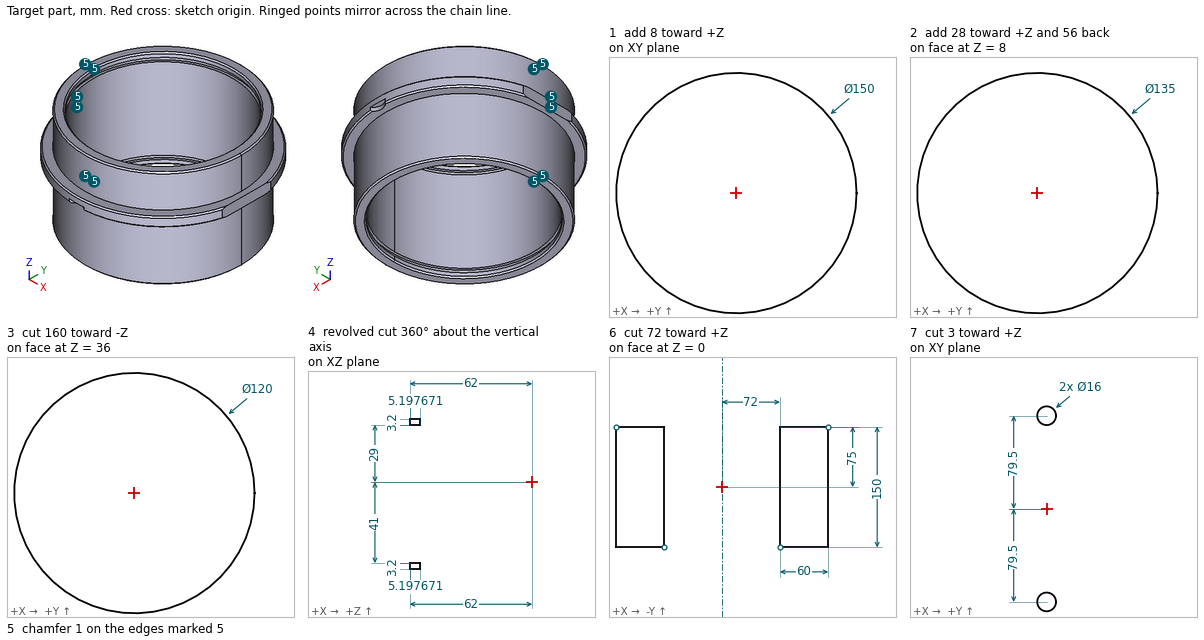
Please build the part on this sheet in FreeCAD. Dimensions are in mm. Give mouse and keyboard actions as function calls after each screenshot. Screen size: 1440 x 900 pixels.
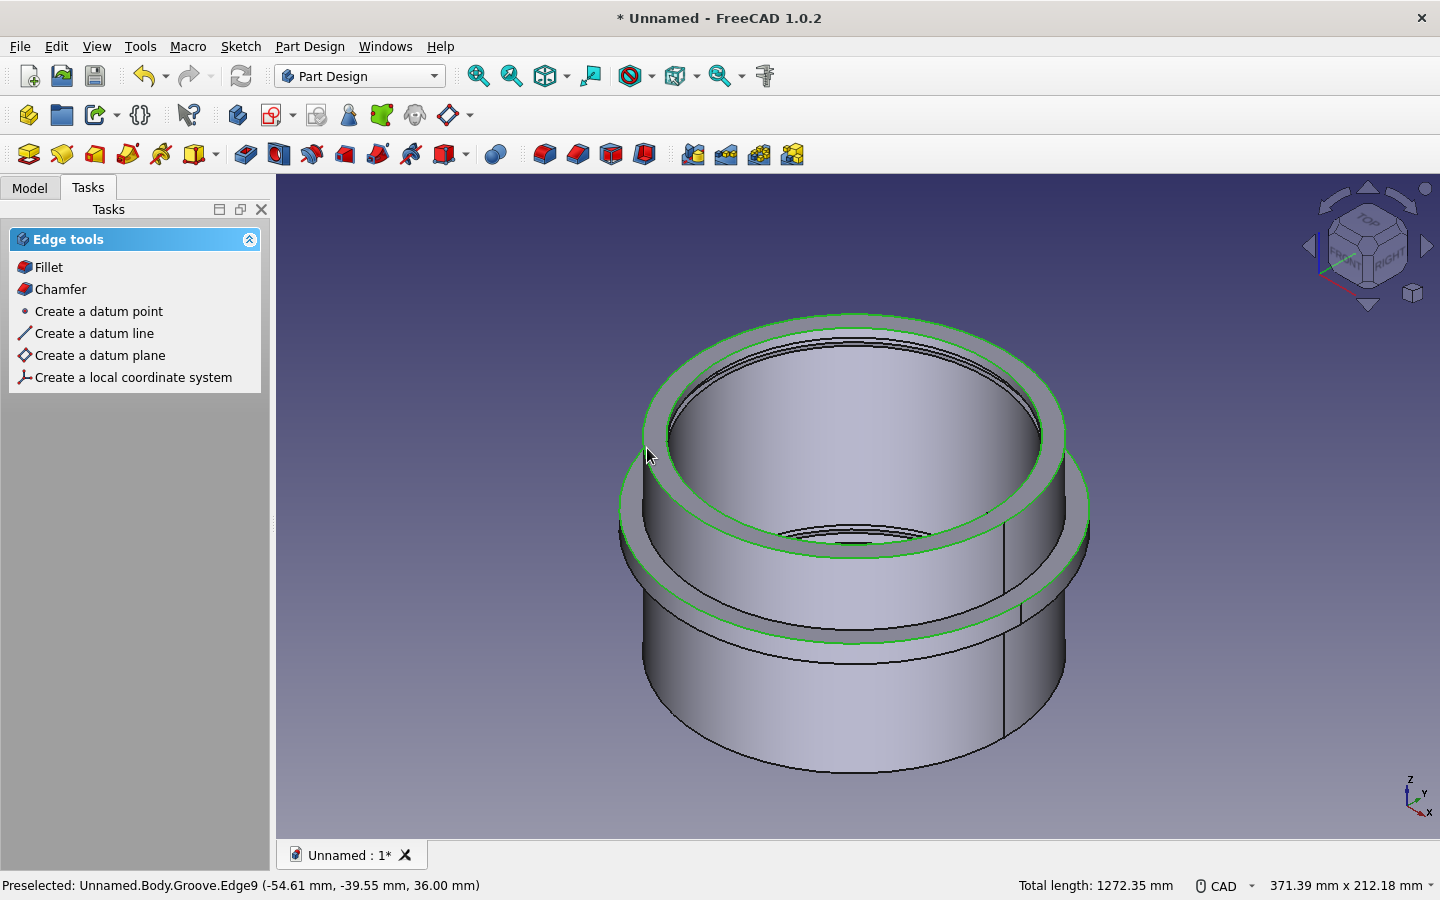
key(v)
key(f)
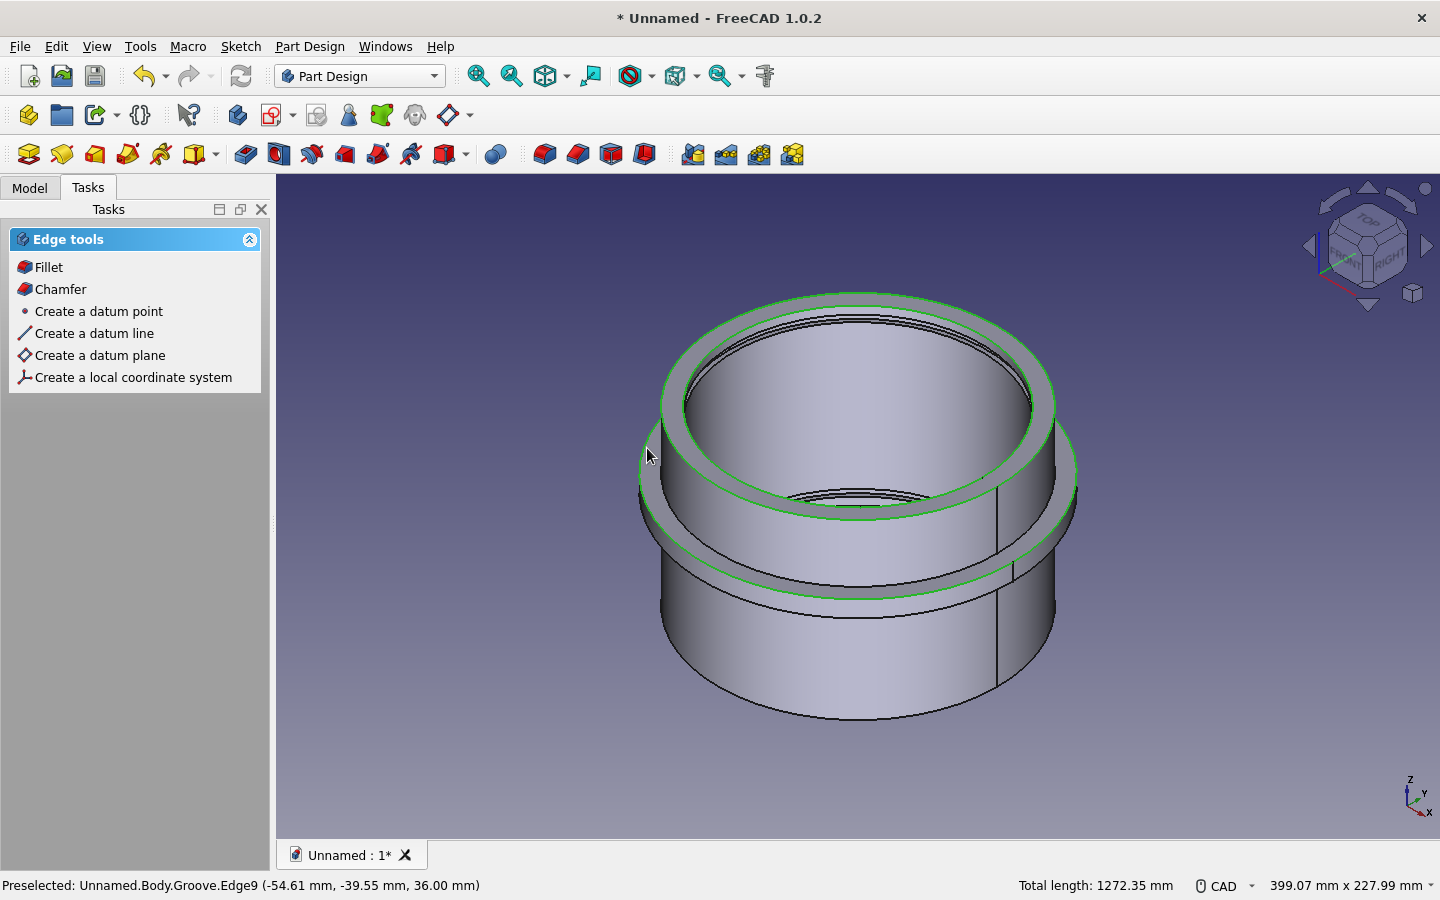
click(663, 549, ctrl)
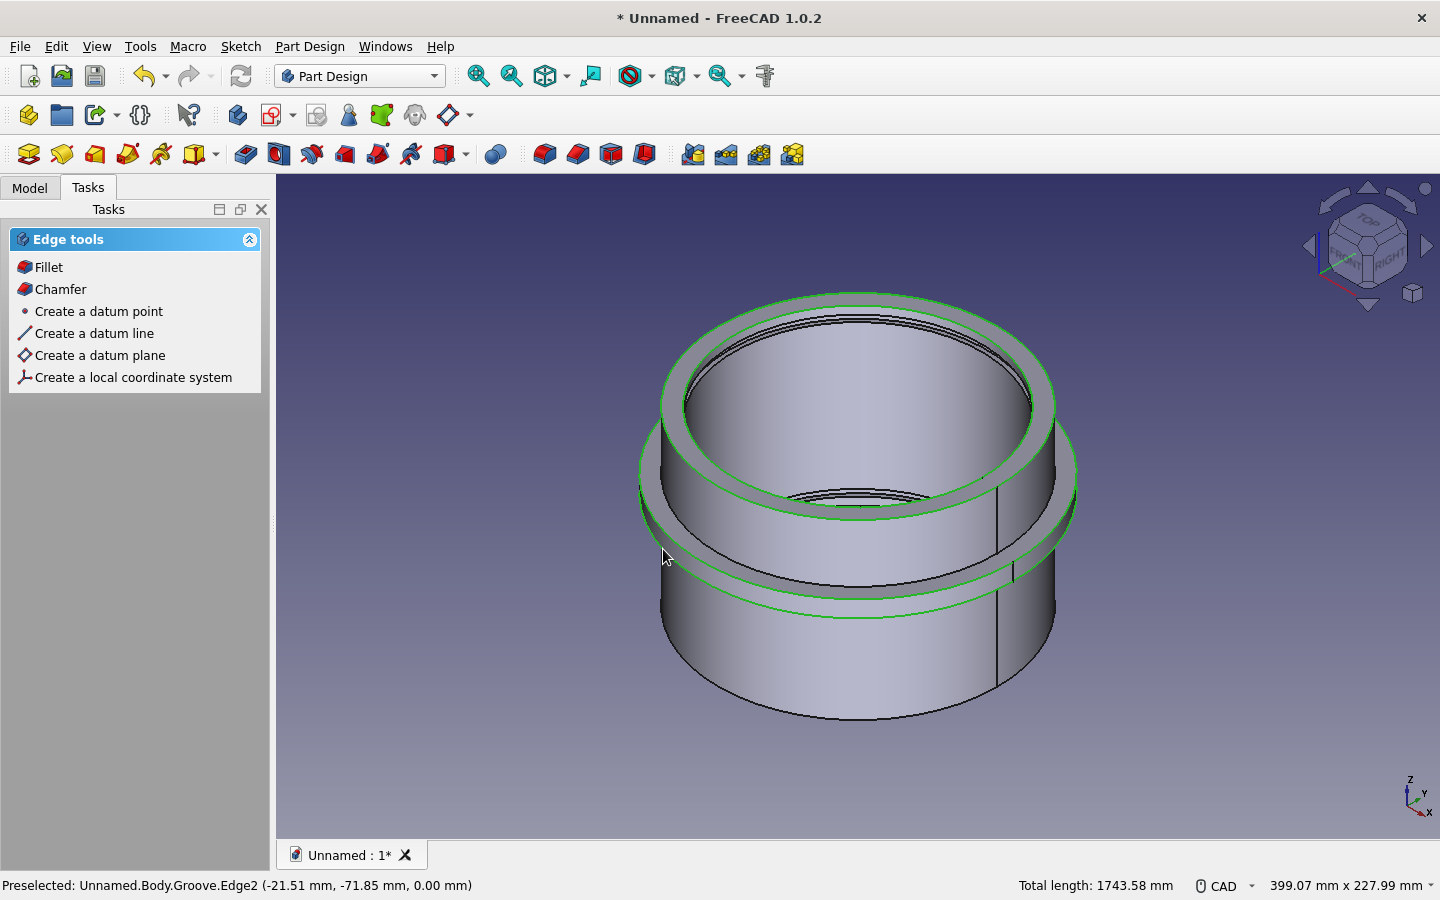
key(2)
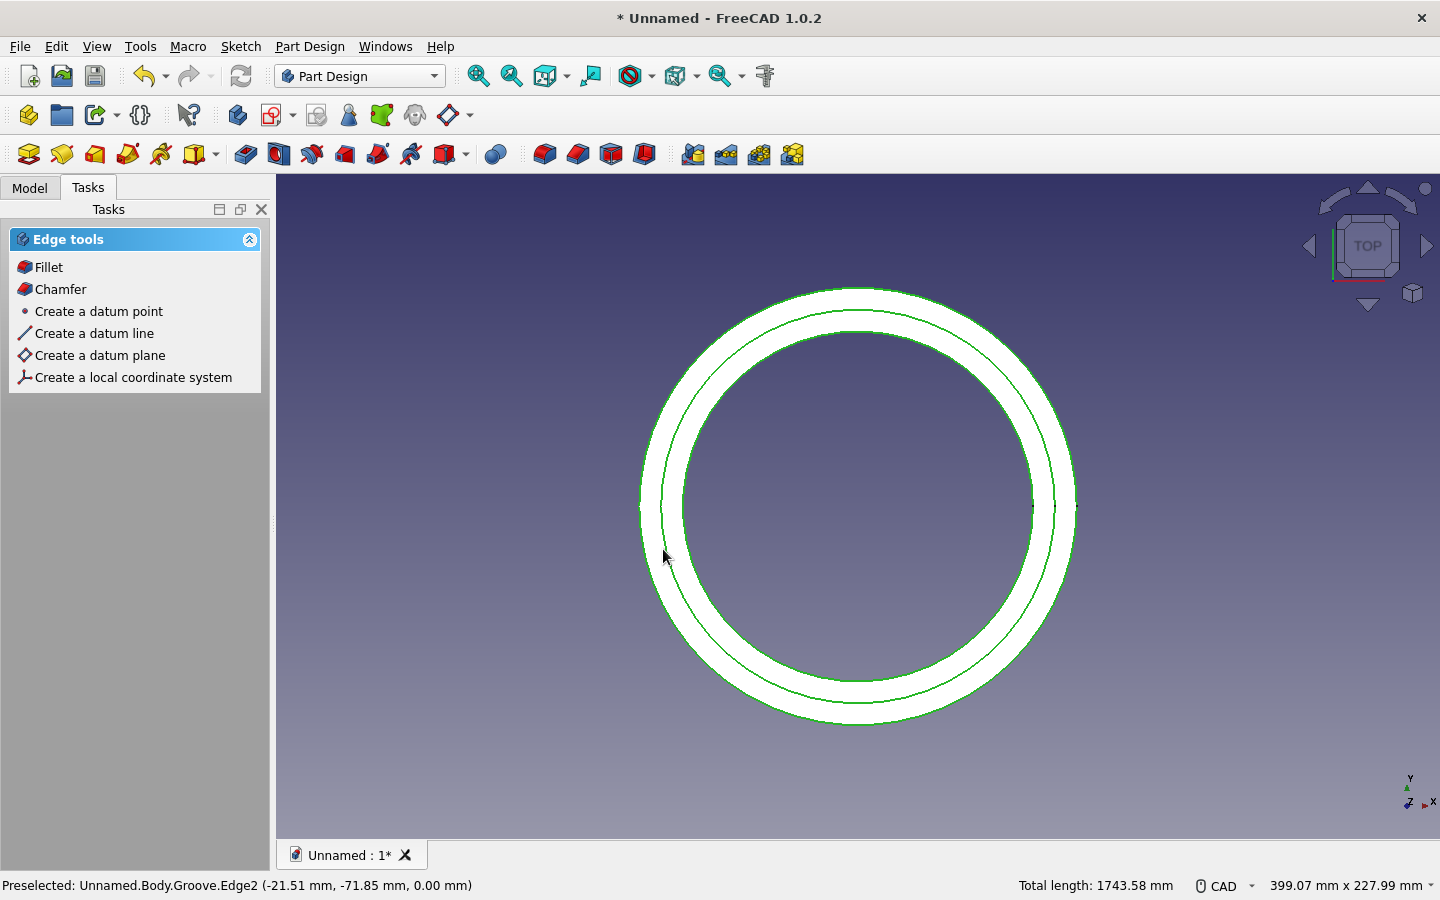
key(1)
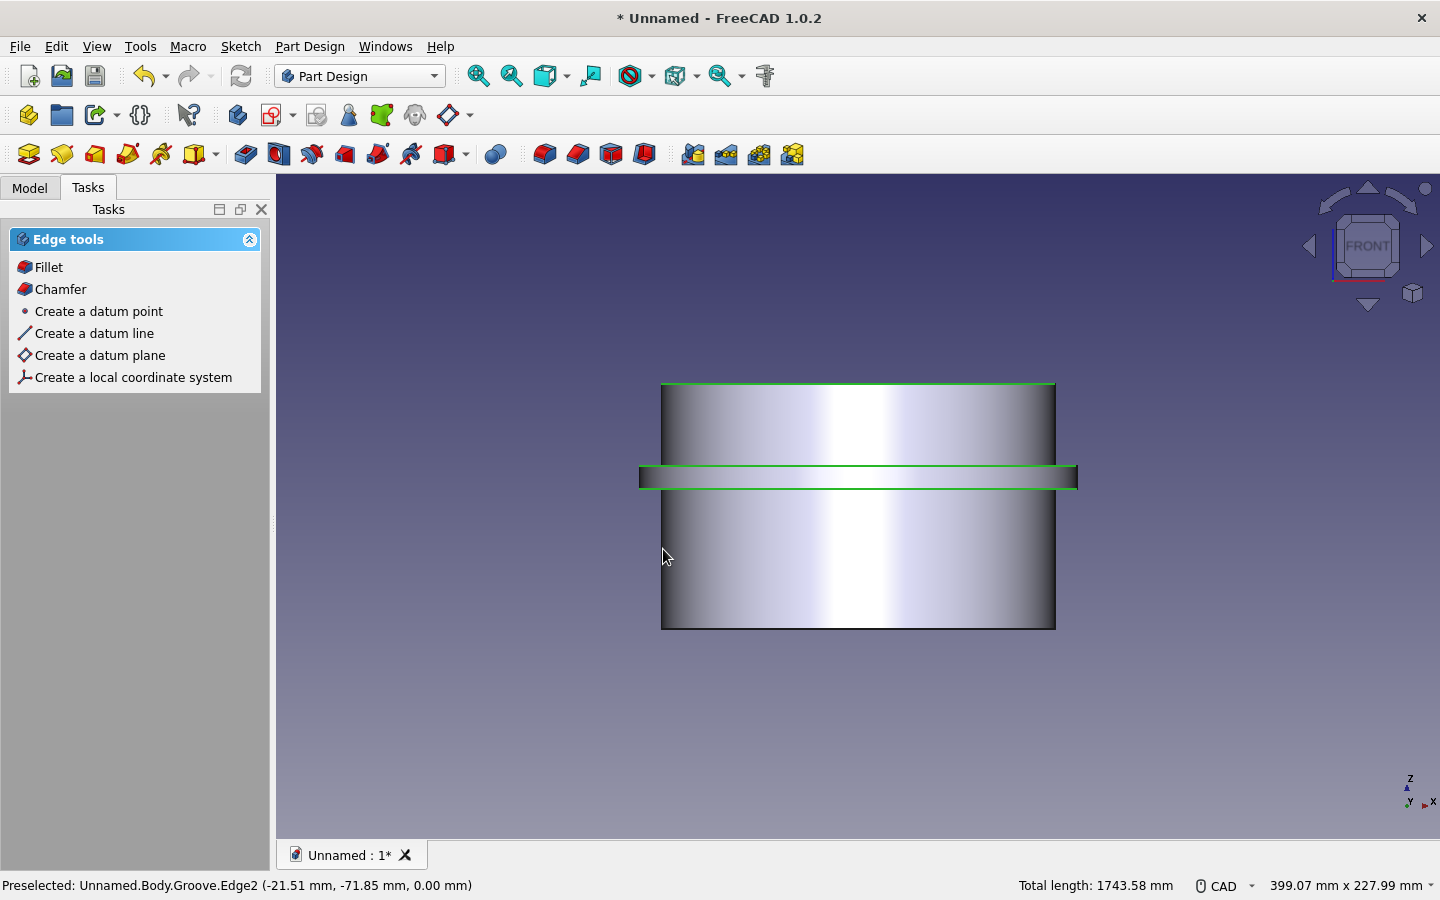
click(479, 76)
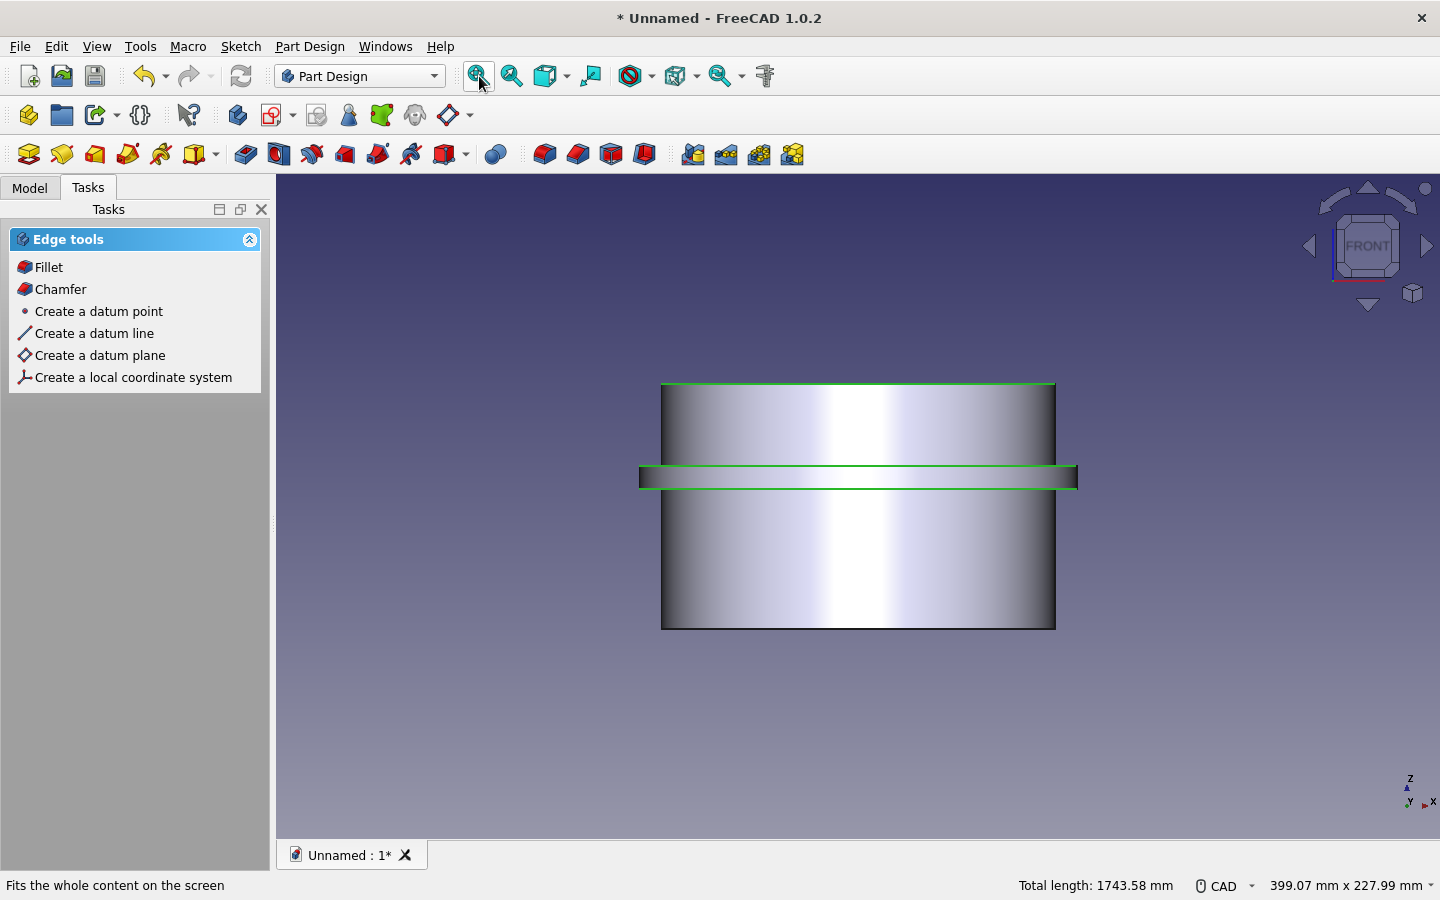
click(699, 628, ctrl)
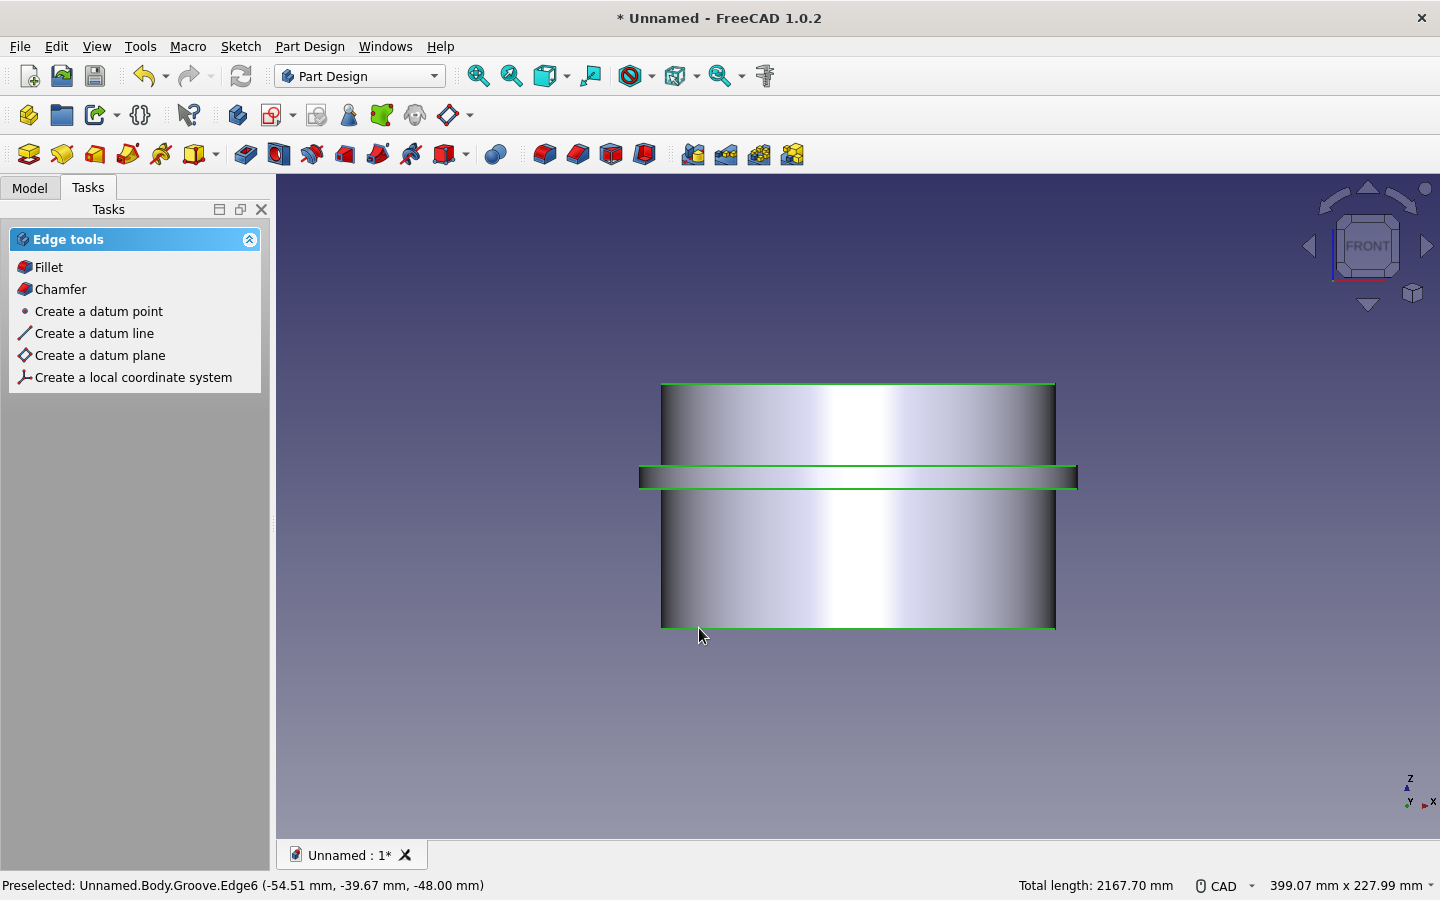
key(3)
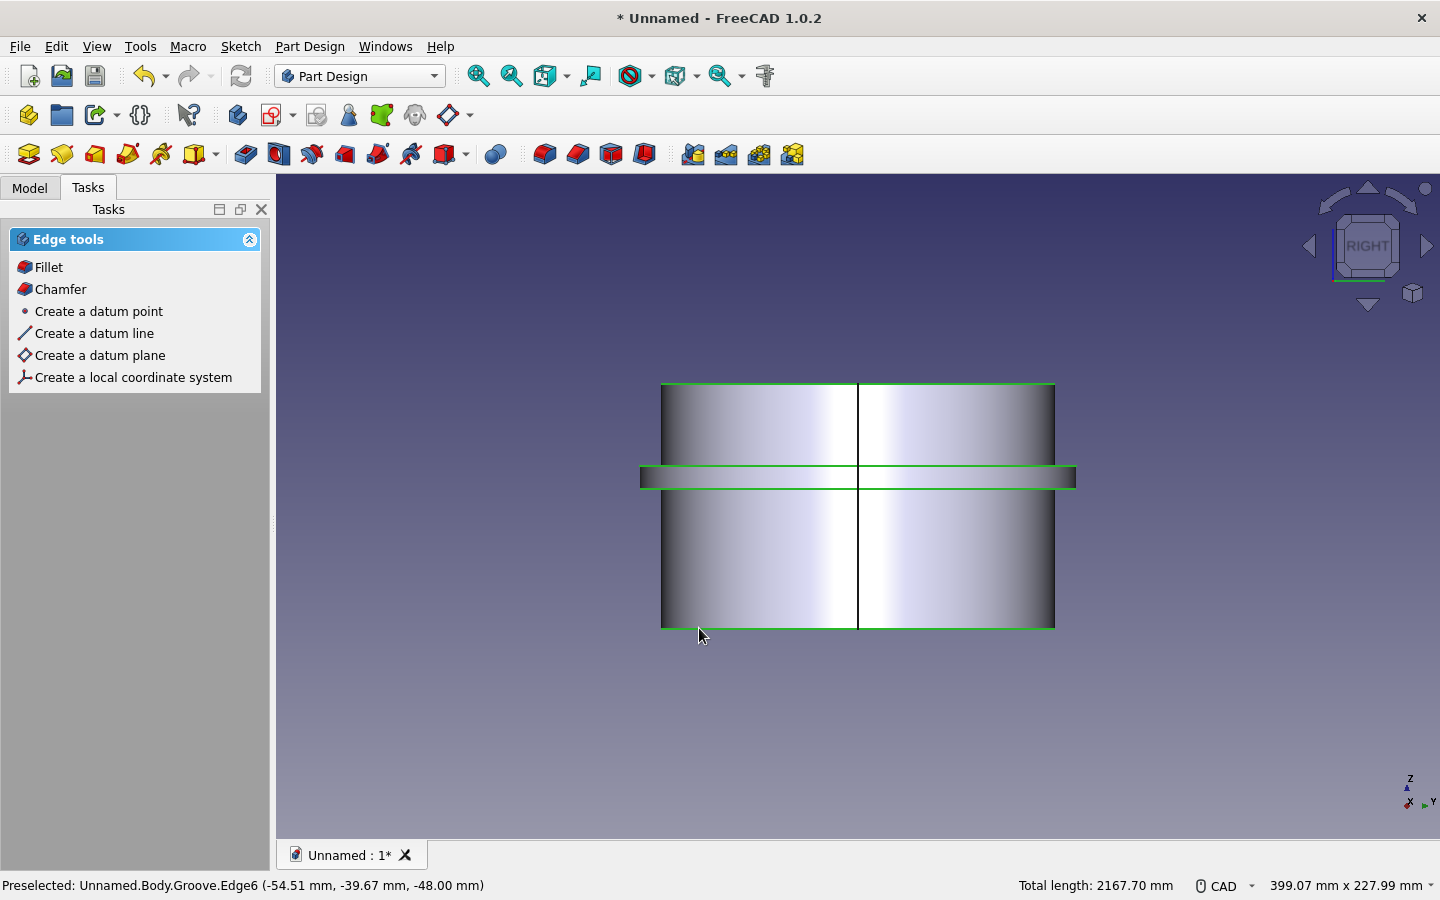
click(479, 76)